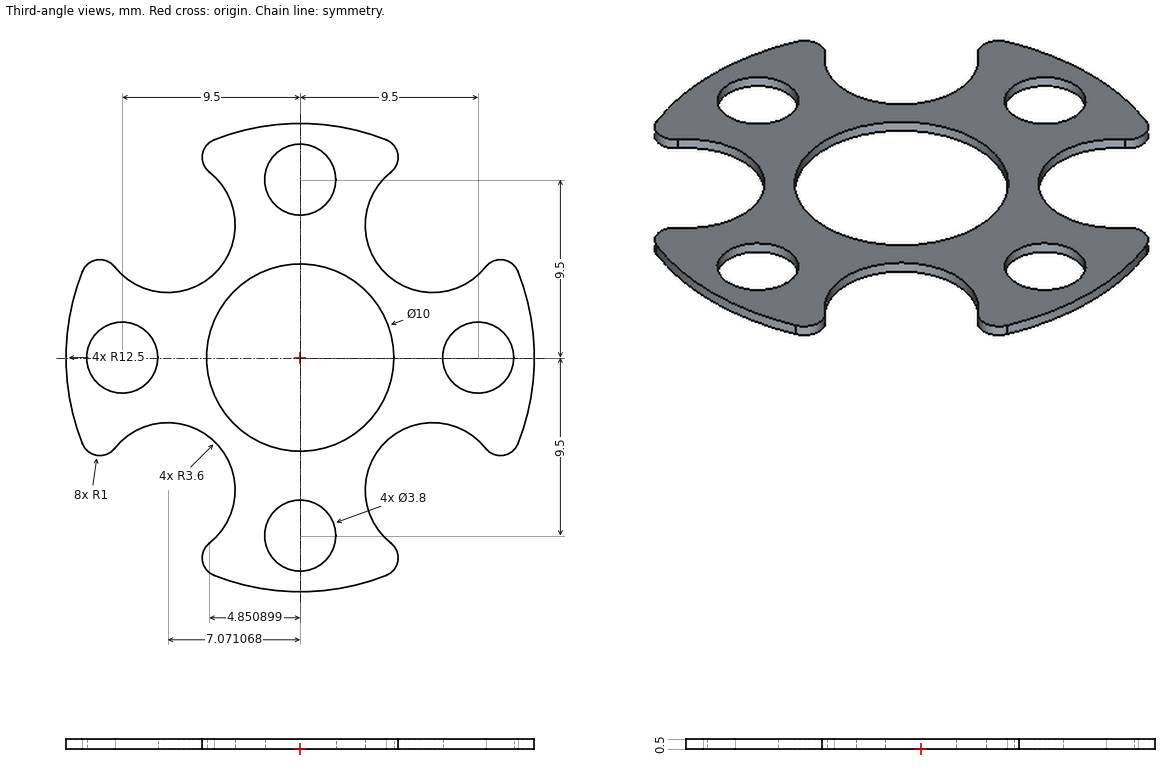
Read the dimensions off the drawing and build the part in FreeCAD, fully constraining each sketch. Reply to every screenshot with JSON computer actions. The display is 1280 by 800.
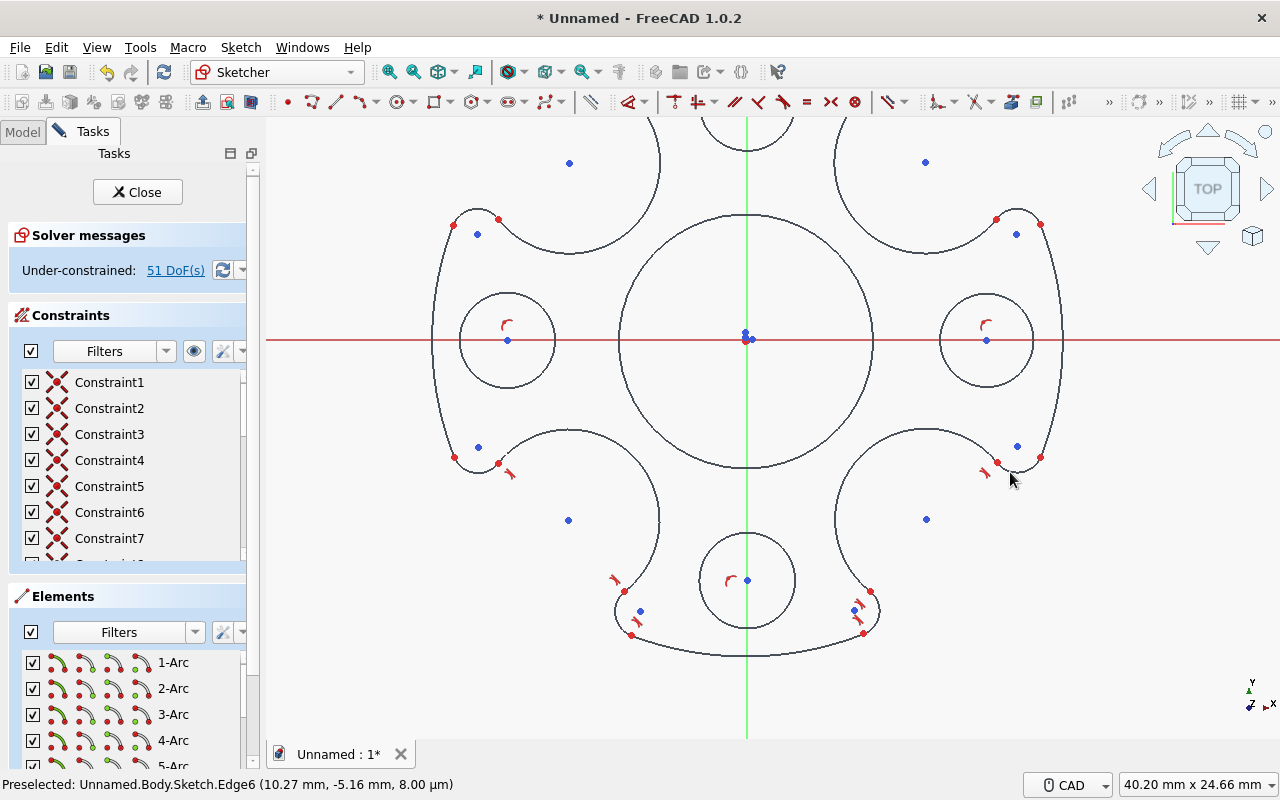
{"action": "left_click", "coordinate": [1010, 472]}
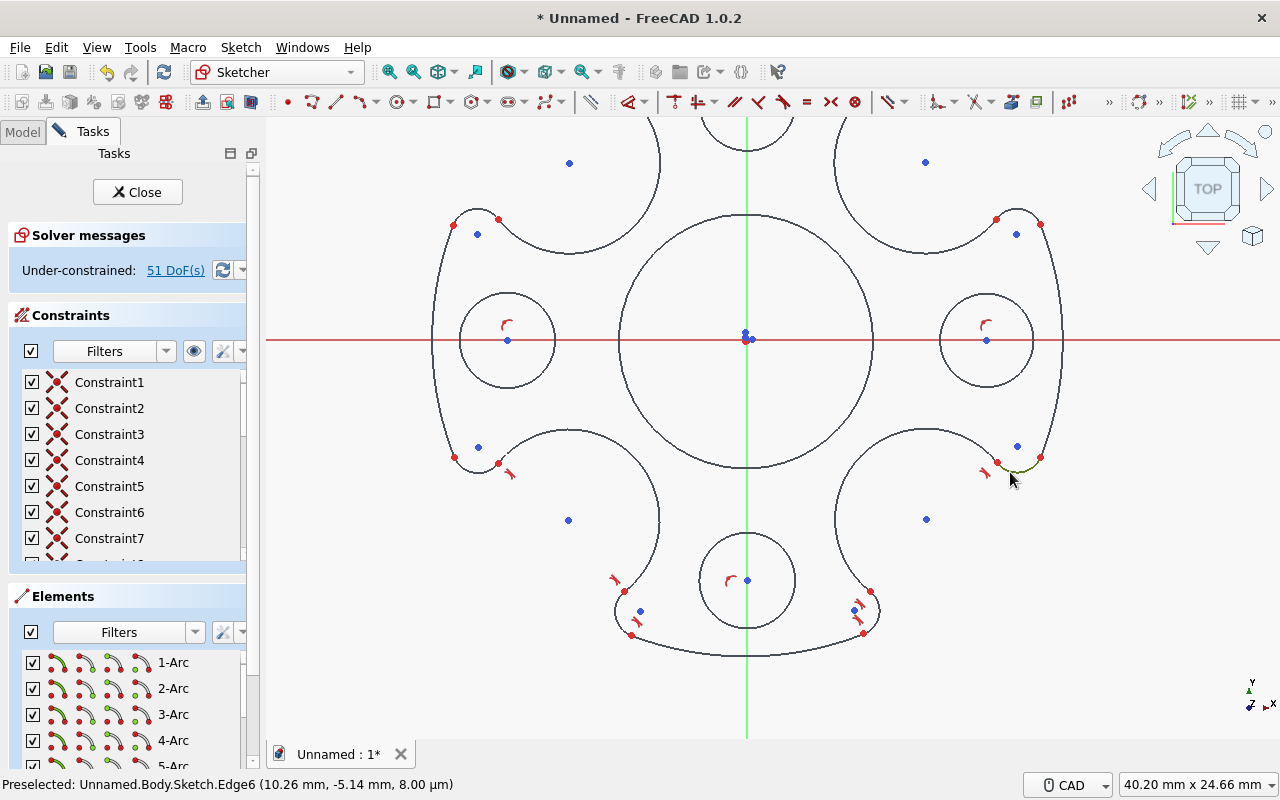
{"action": "left_click", "coordinate": [1059, 389]}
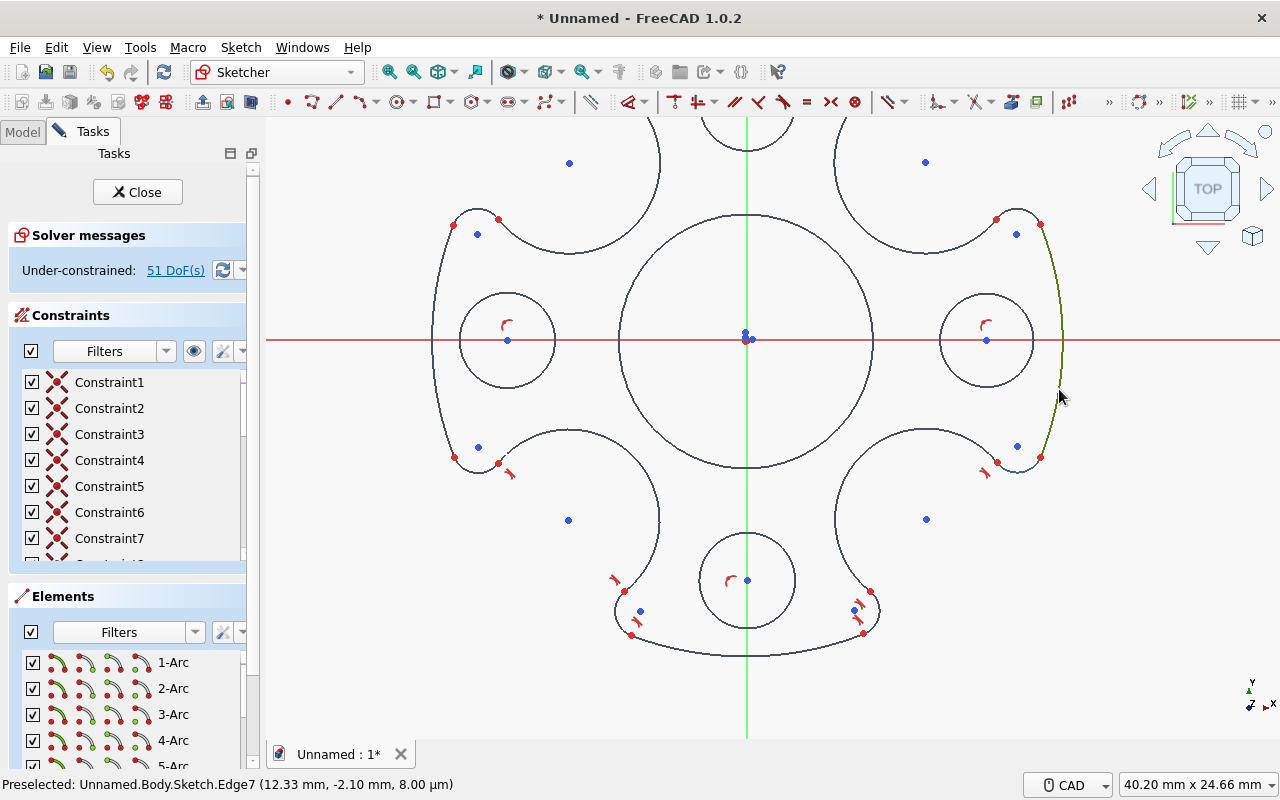
{"action": "key", "text": "t"}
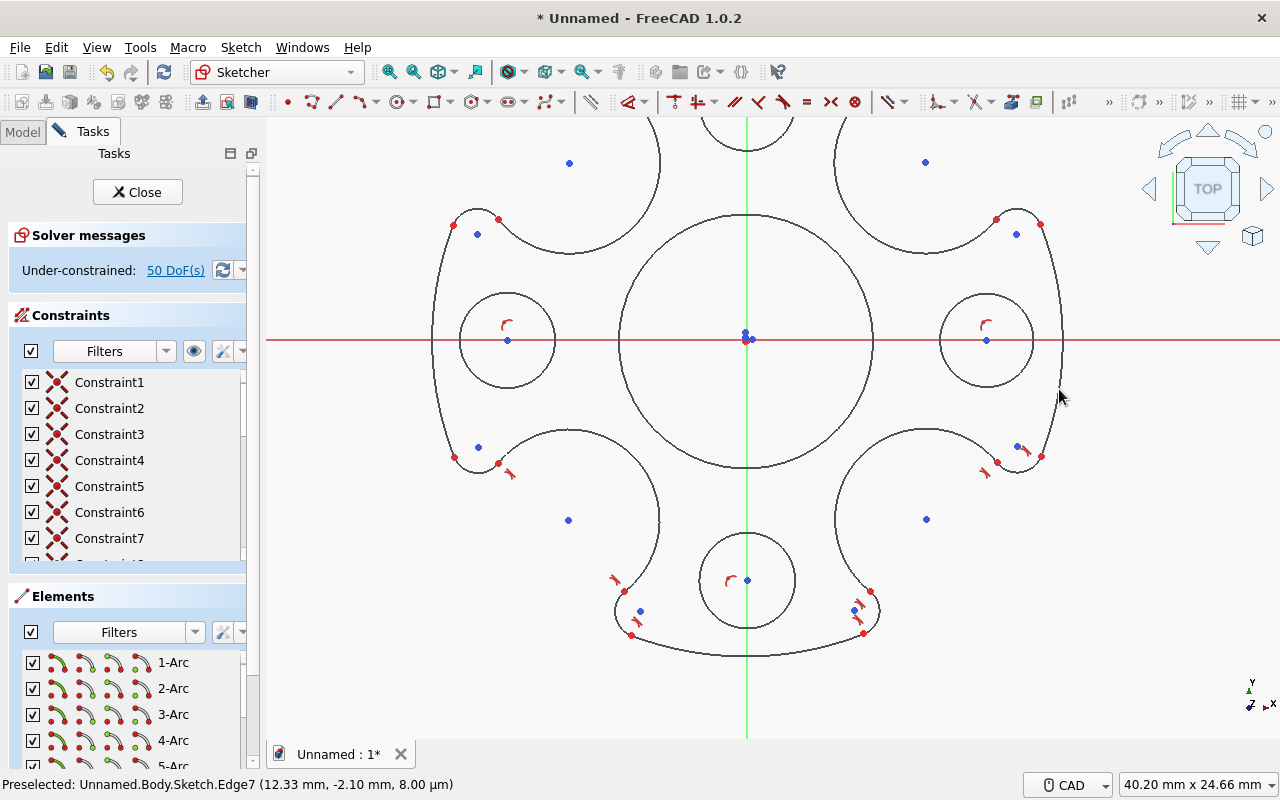
{"action": "left_click", "coordinate": [1059, 388]}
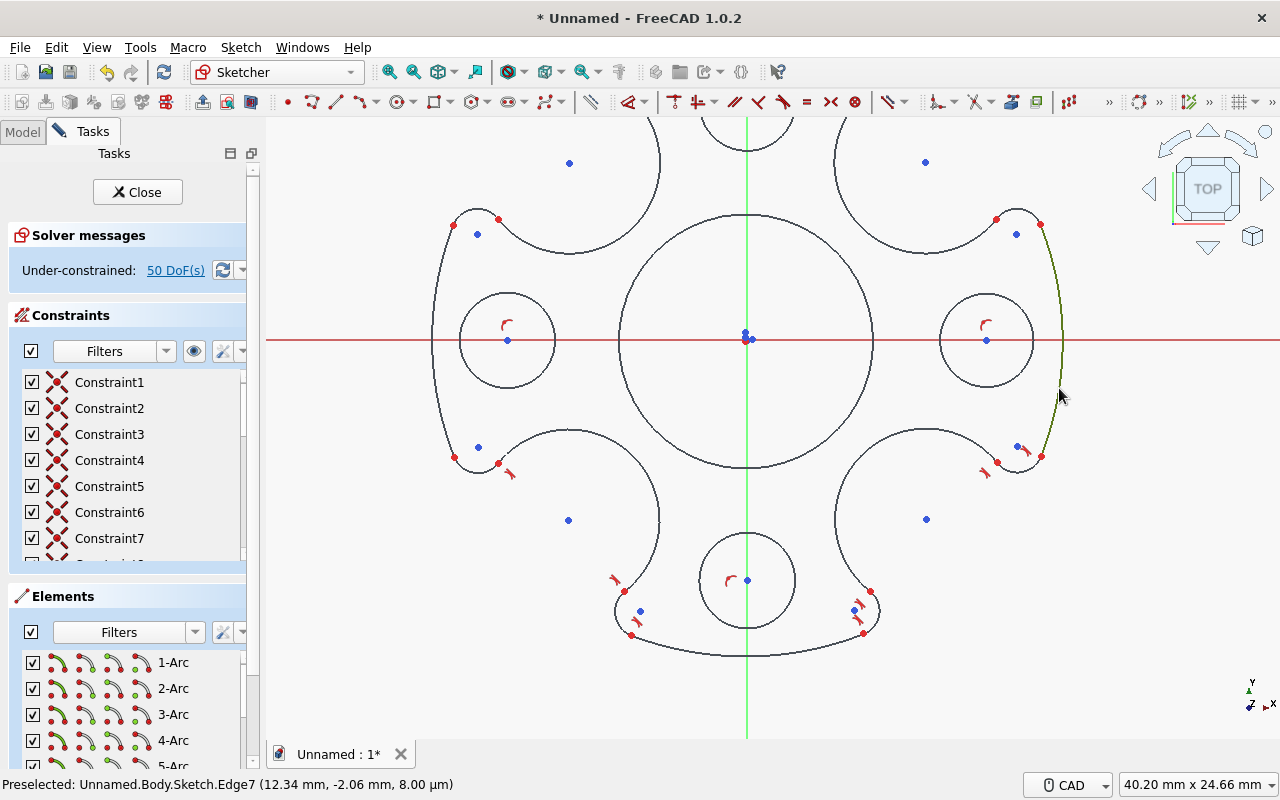
{"action": "left_click", "coordinate": [1030, 213]}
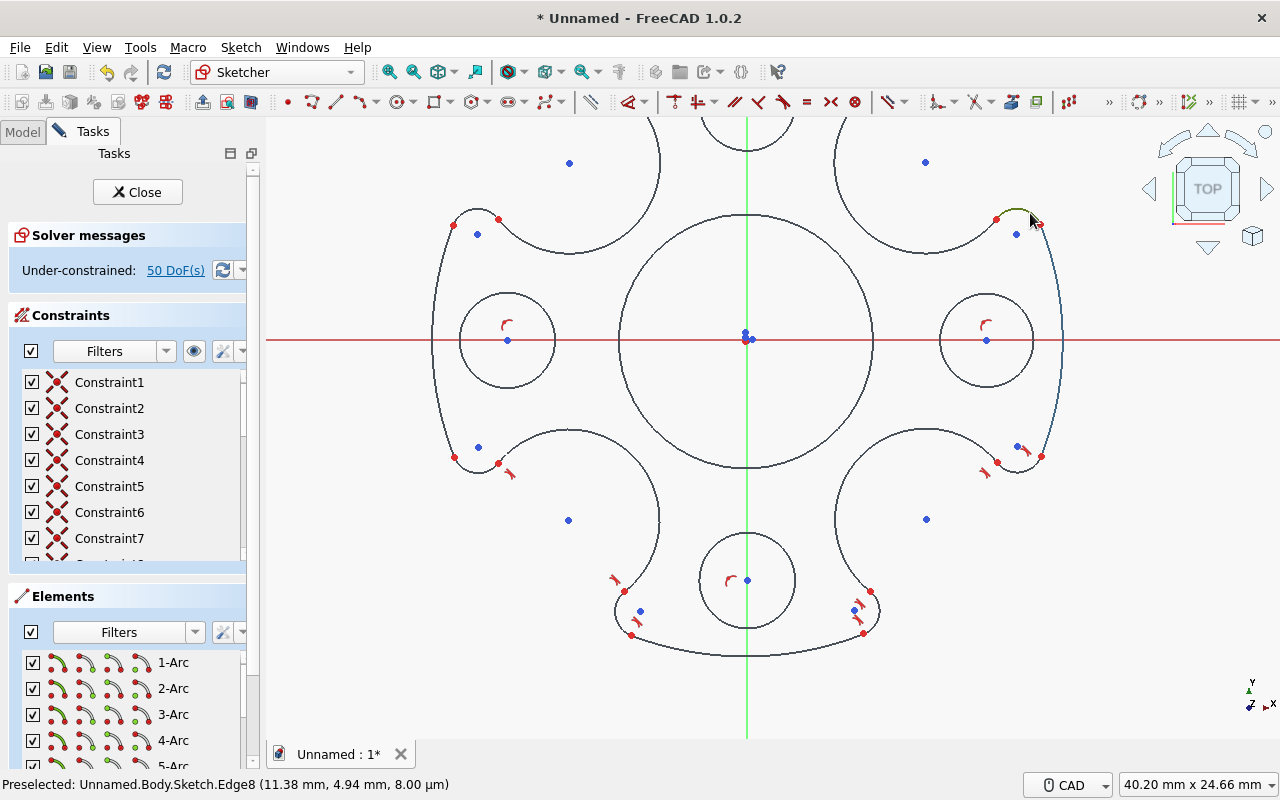
{"action": "key", "text": "t"}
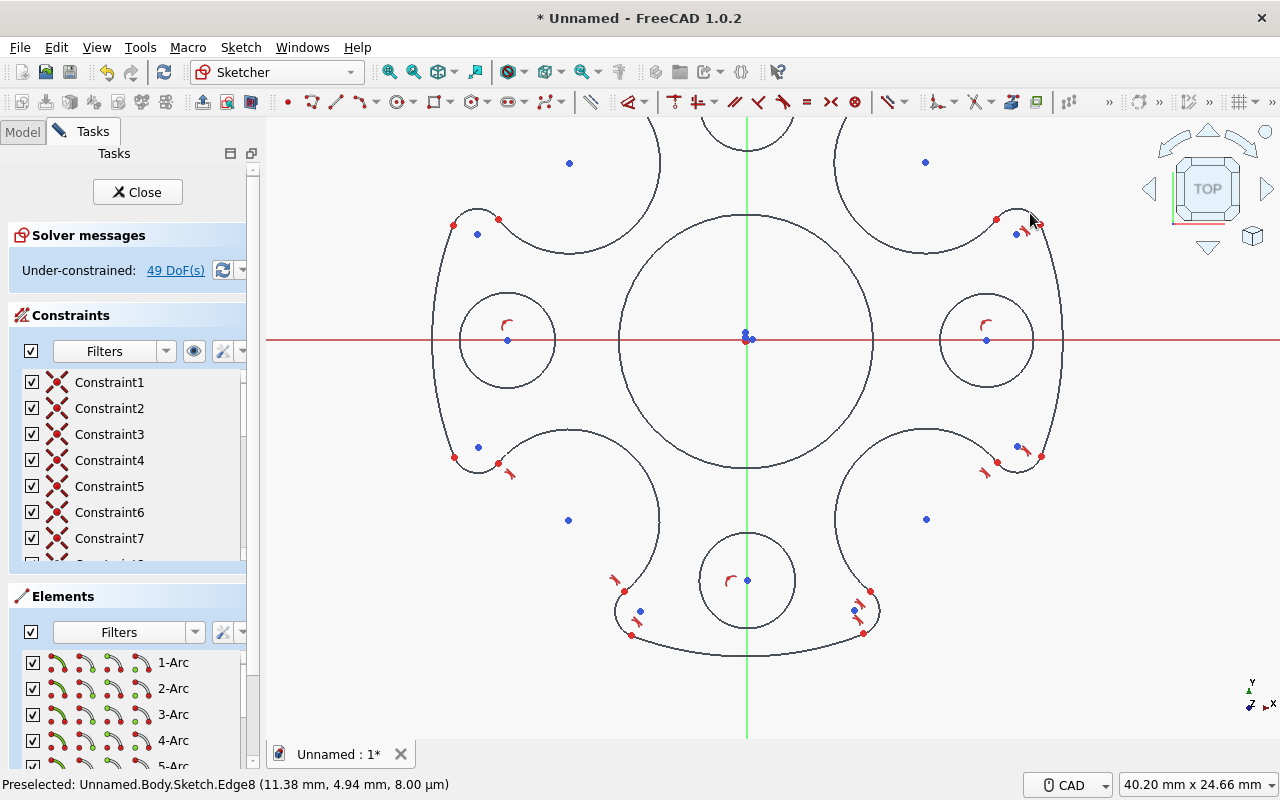
{"action": "left_click", "coordinate": [1030, 213]}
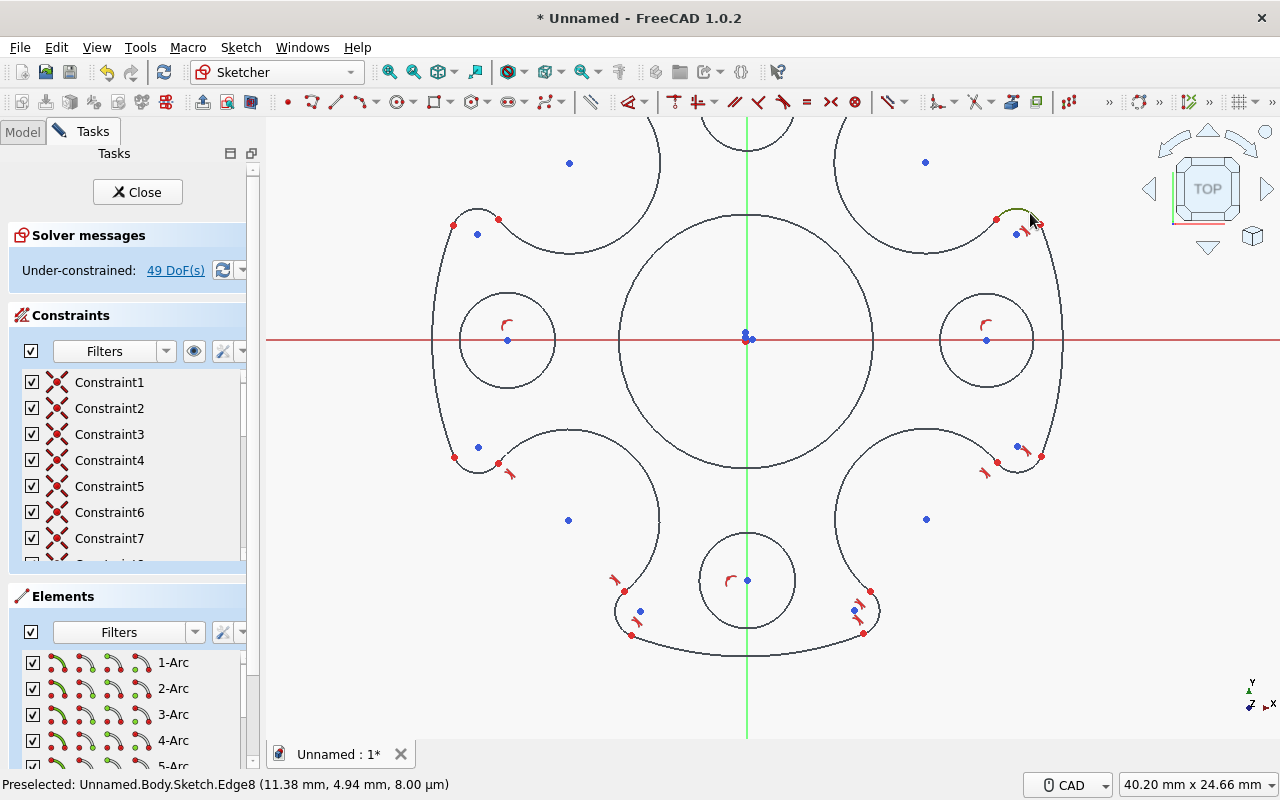
{"action": "left_click", "coordinate": [835, 172]}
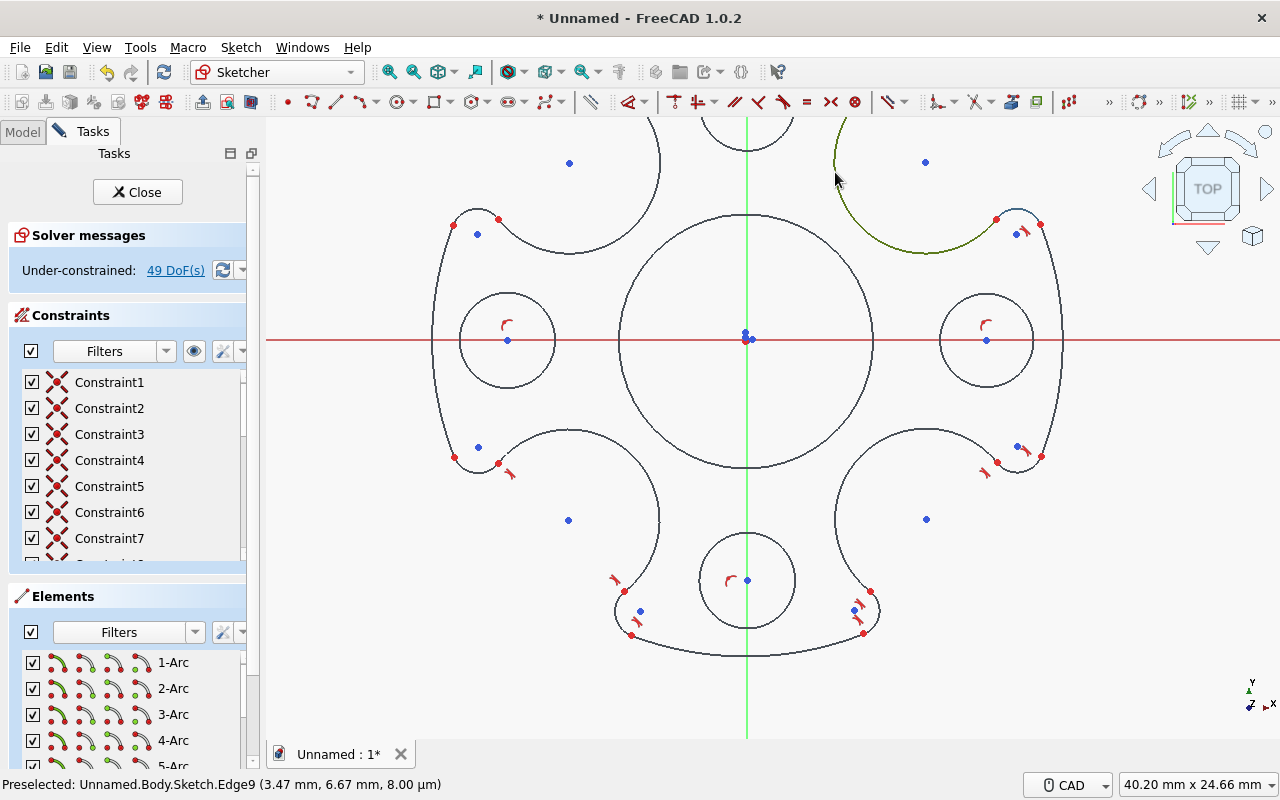
{"action": "key", "text": "t"}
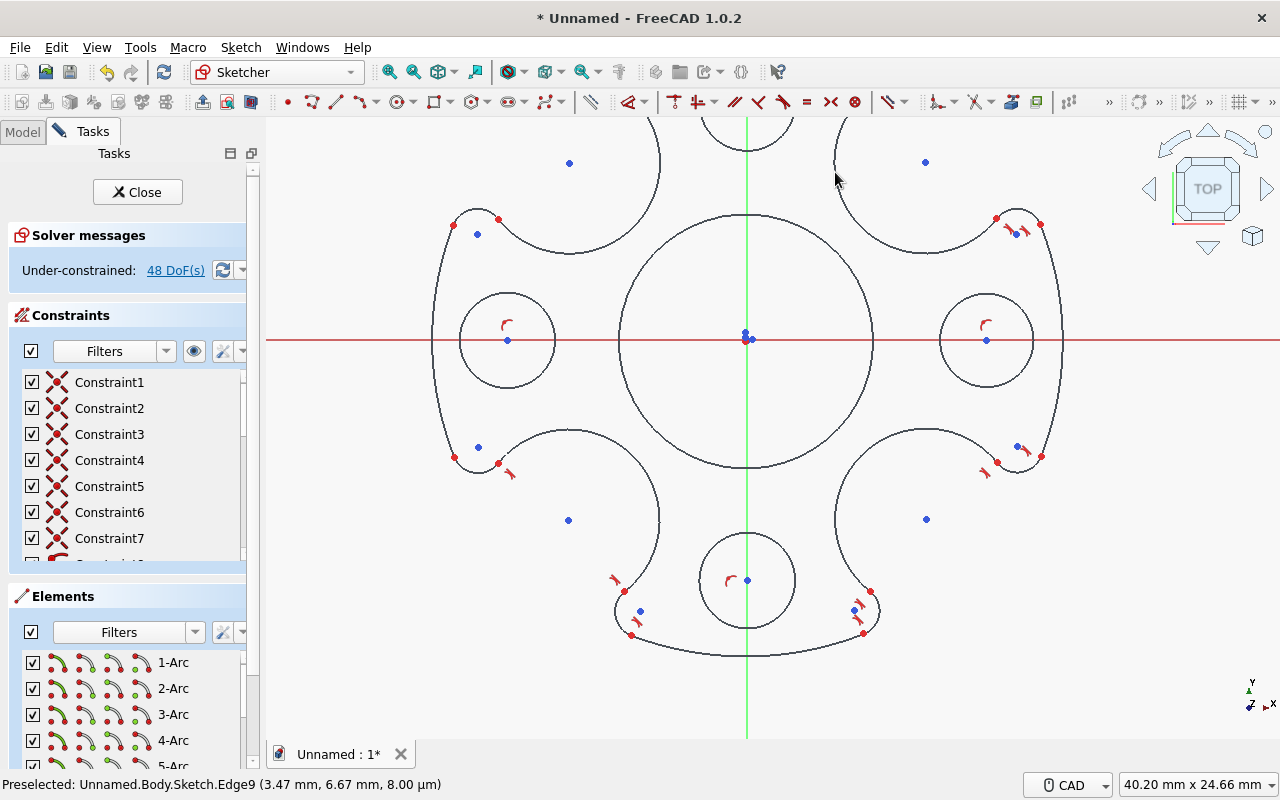
{"action": "left_click", "coordinate": [835, 173]}